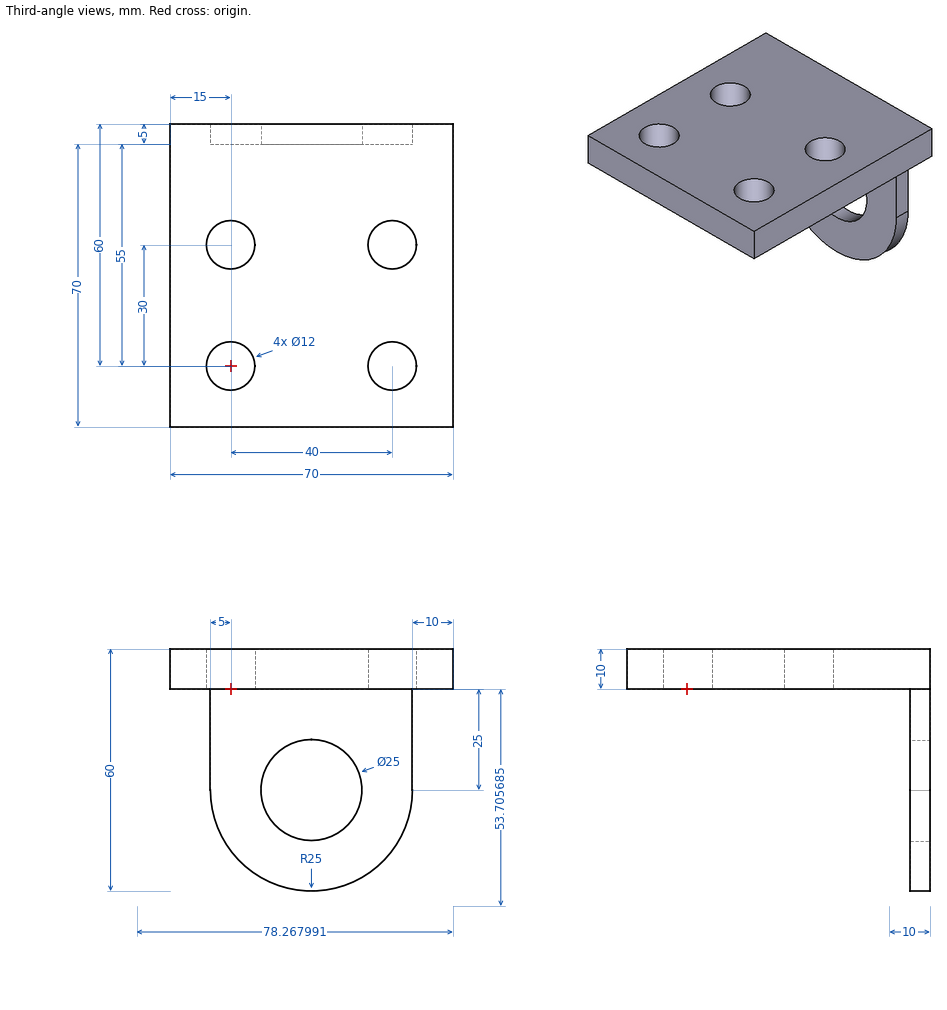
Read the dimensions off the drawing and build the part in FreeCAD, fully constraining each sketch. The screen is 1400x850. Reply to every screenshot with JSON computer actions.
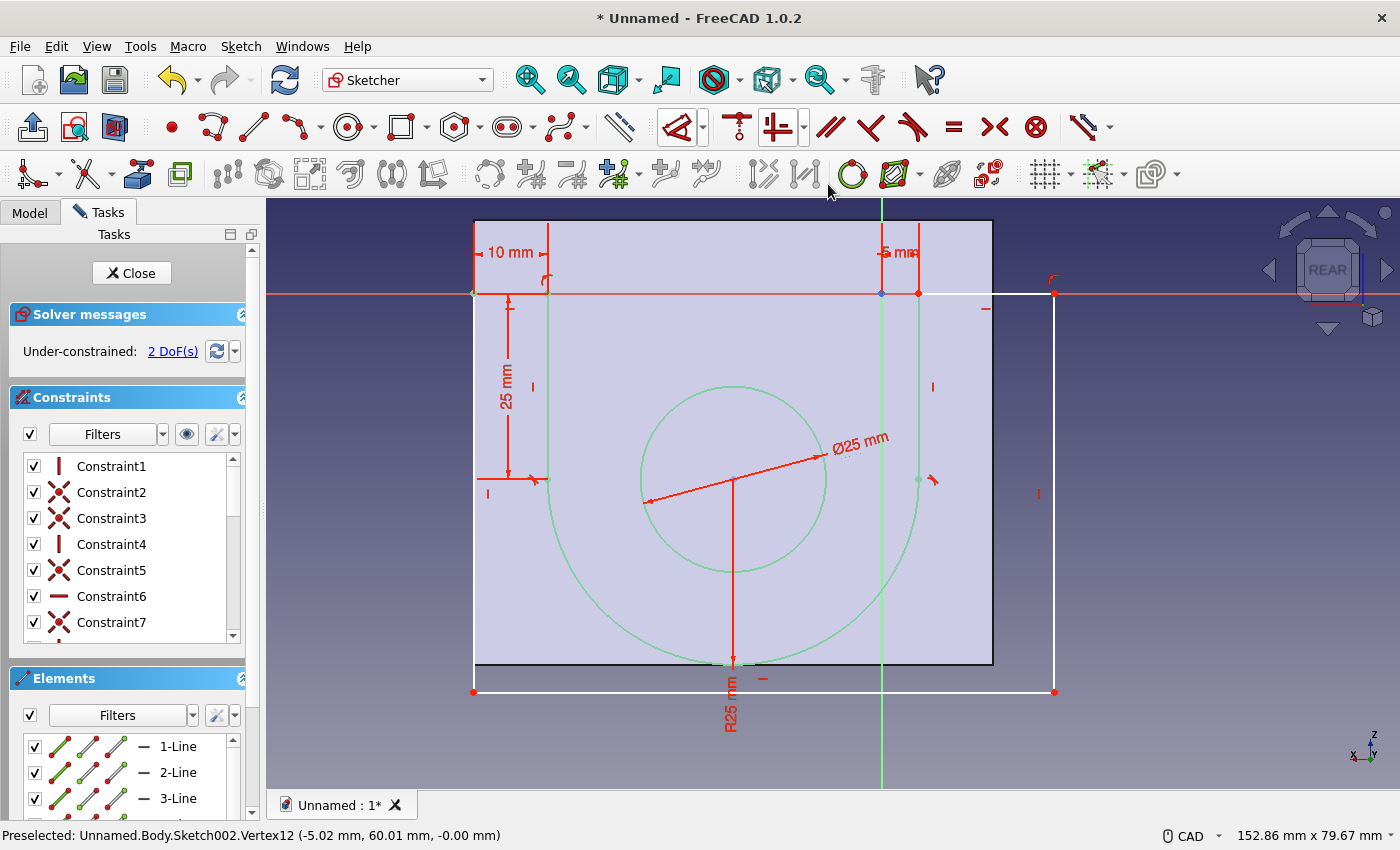
{"action": "left_click", "coordinate": [474, 414]}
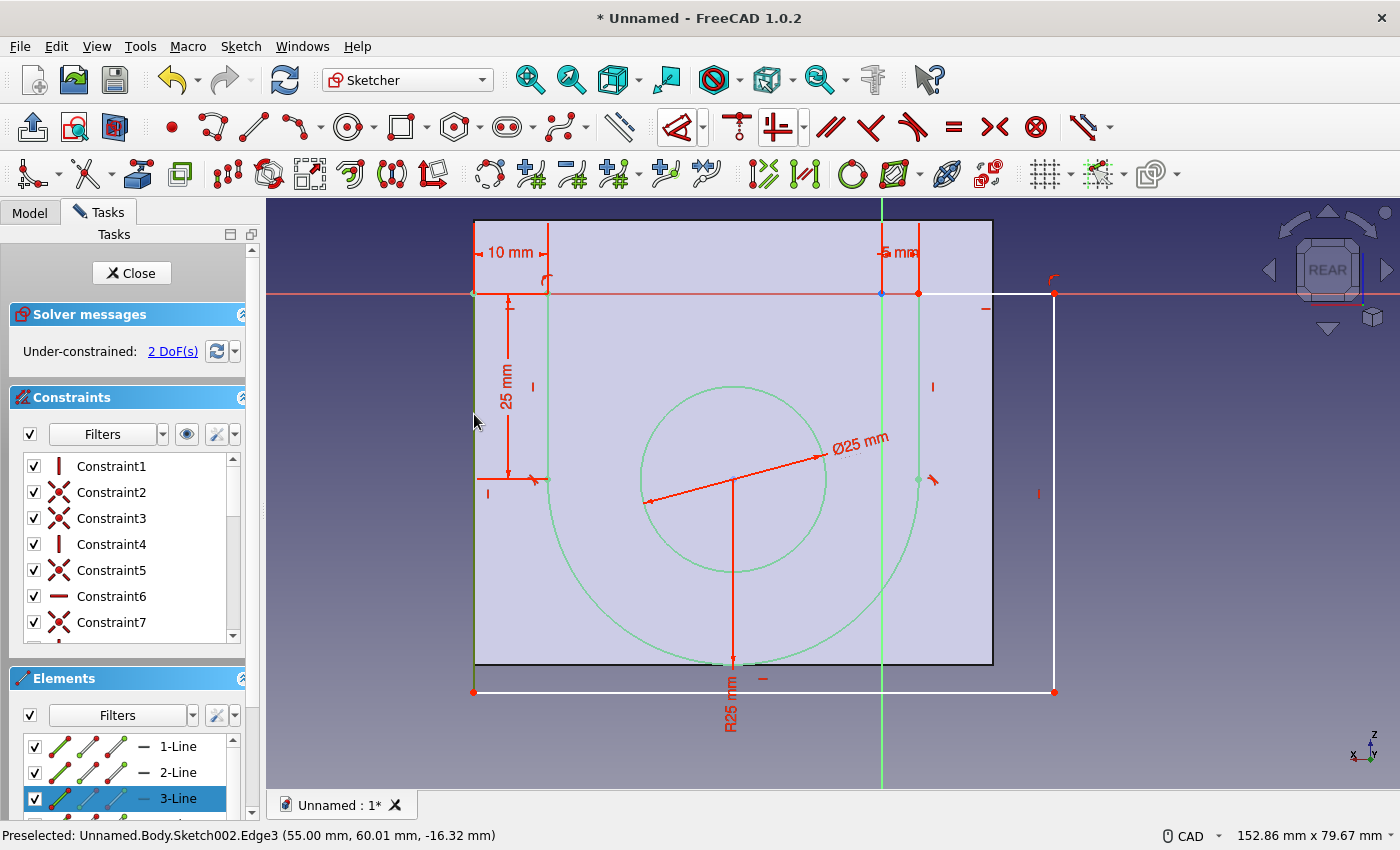
{"action": "key", "text": "i"}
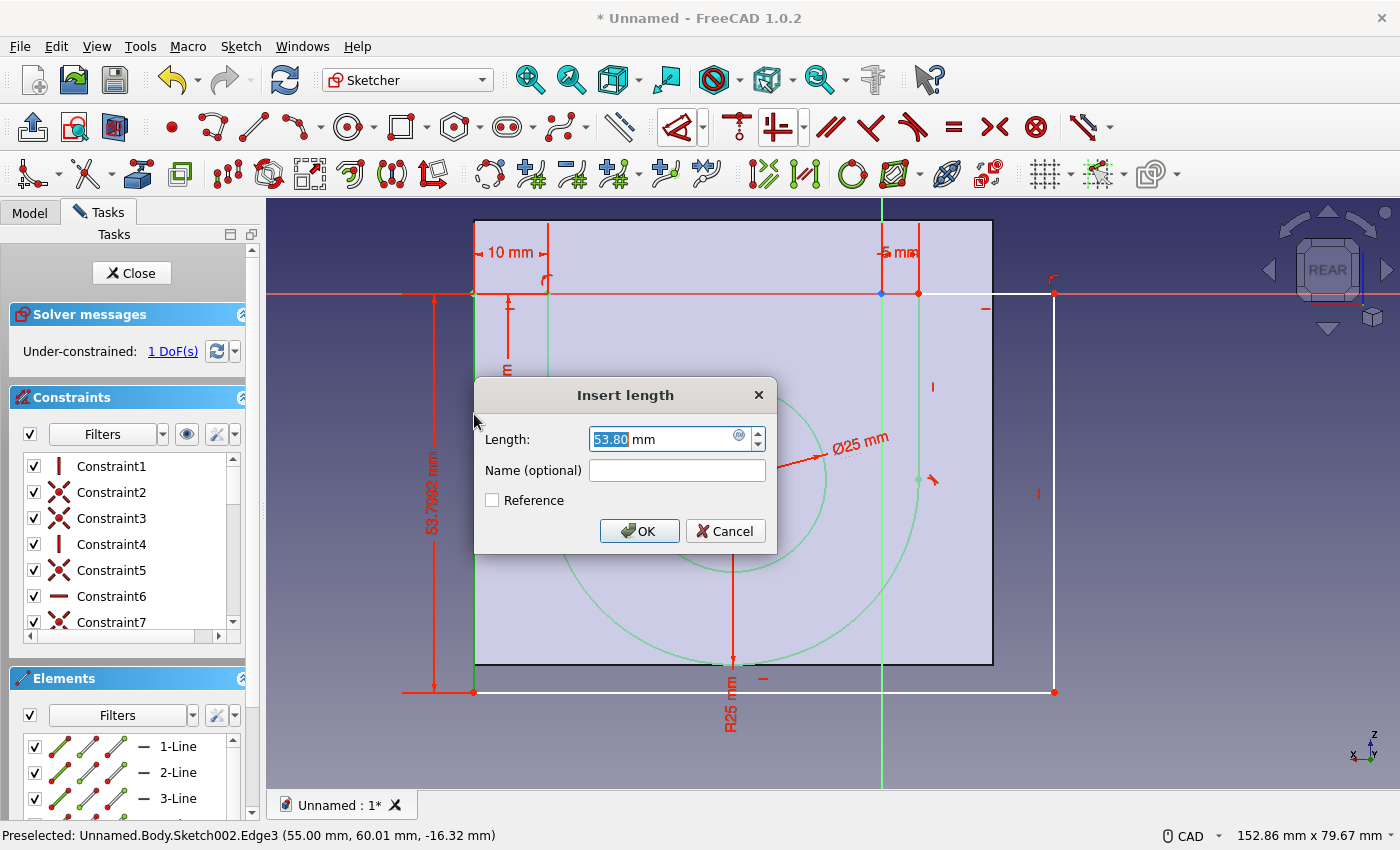
{"action": "type", "text": "53.705685"}
{"action": "key", "text": "Return"}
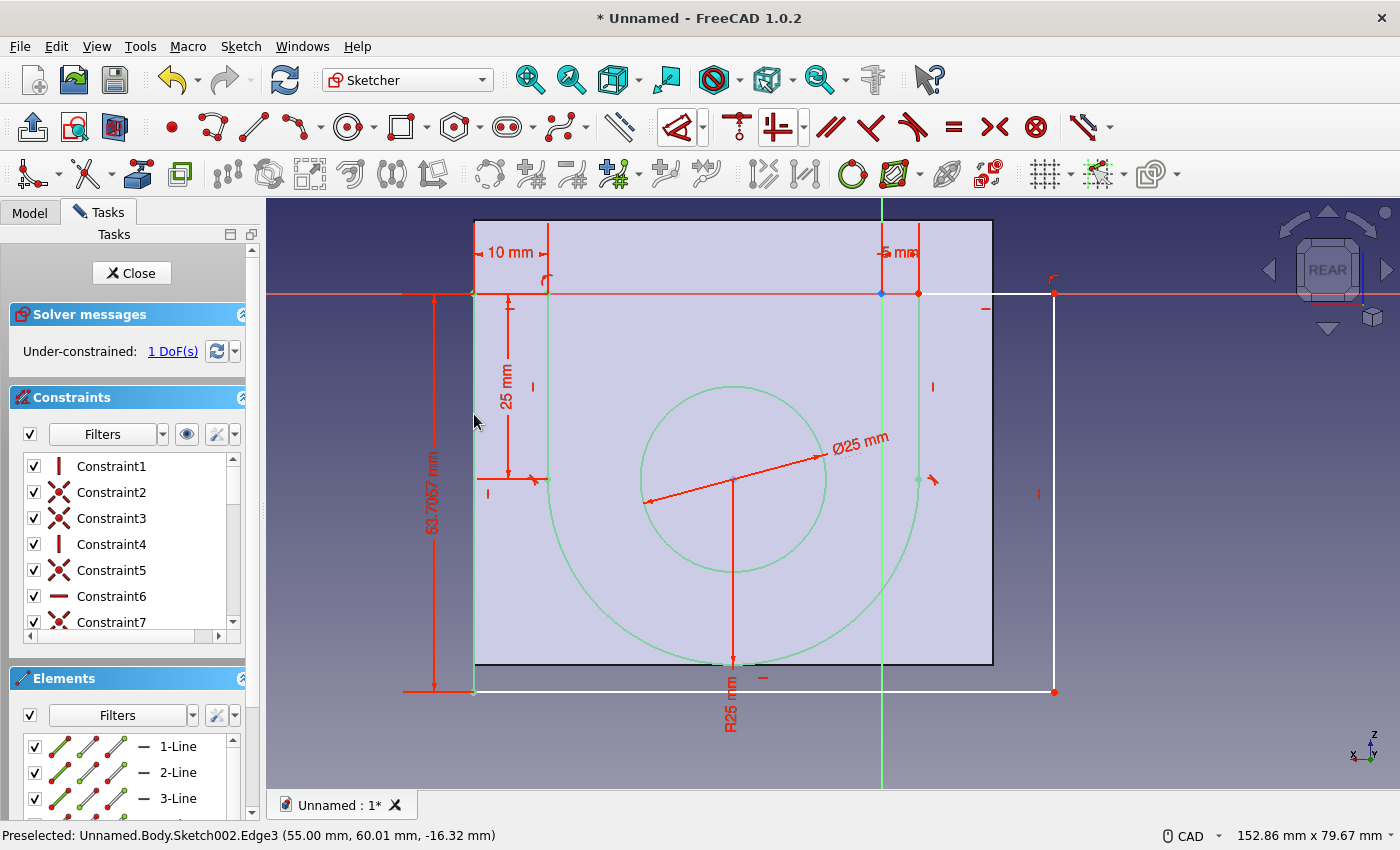
{"action": "left_click", "coordinate": [648, 692]}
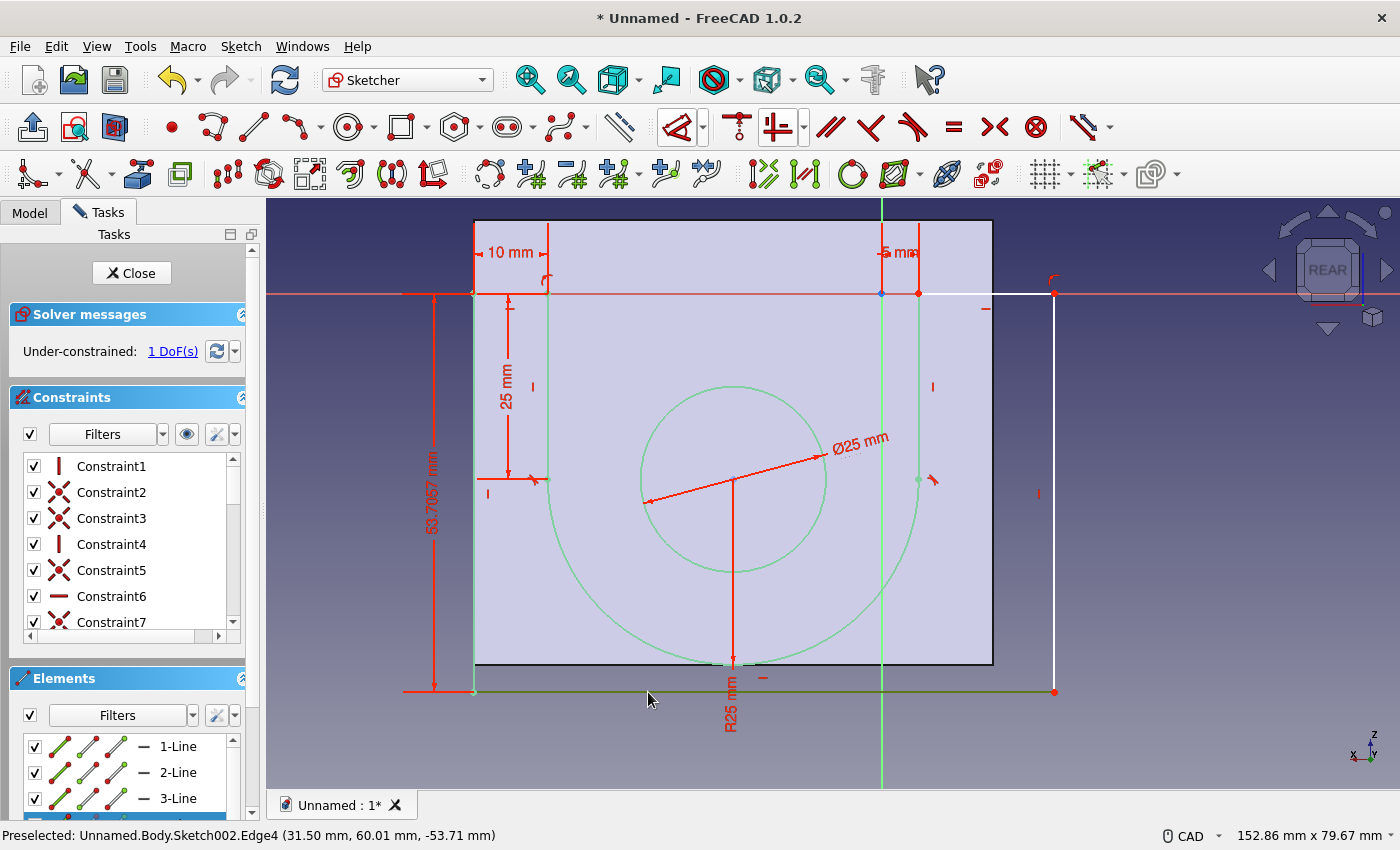
{"action": "key", "text": "l"}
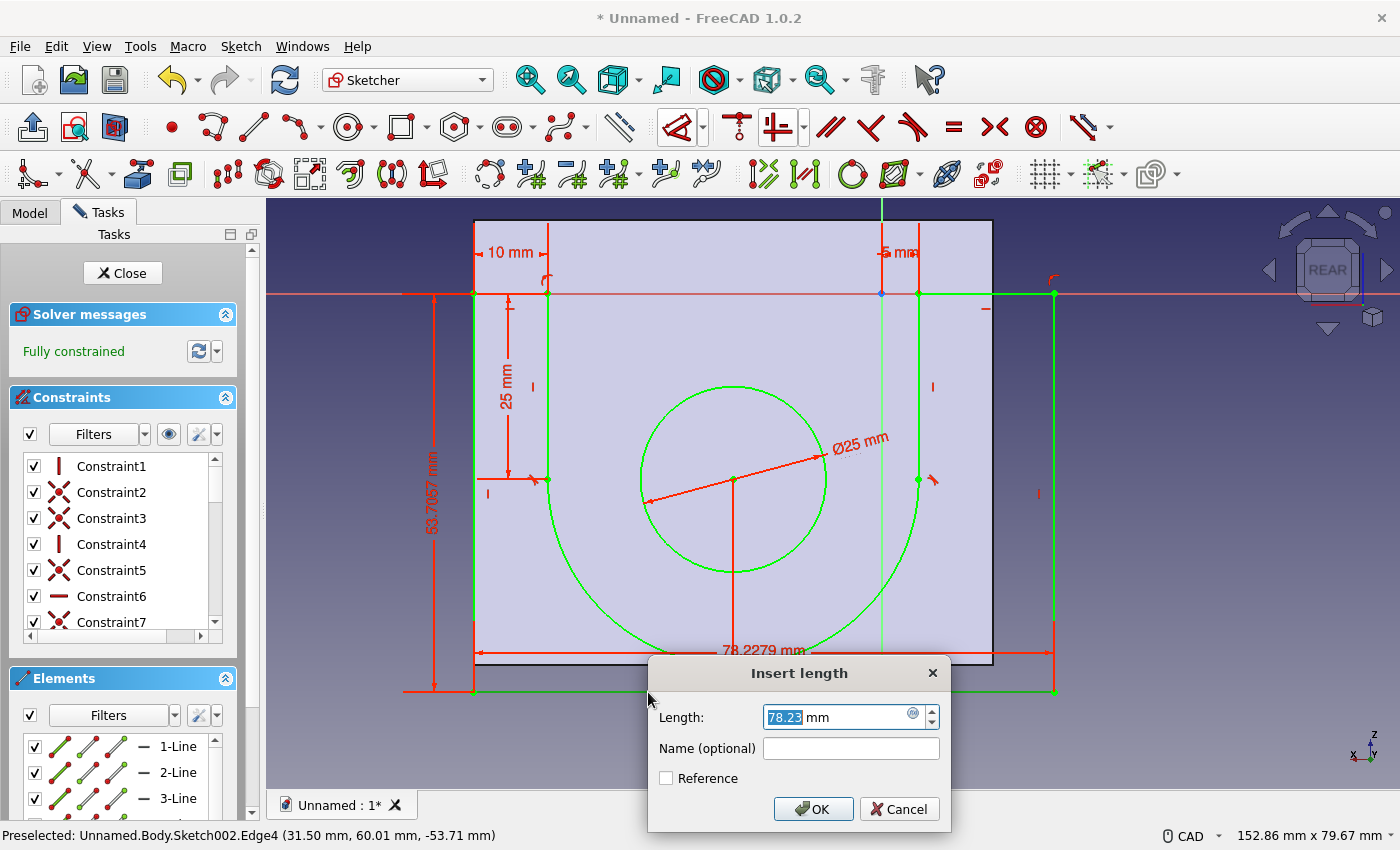
{"action": "type", "text": "78.267991"}
{"action": "key", "text": "Return"}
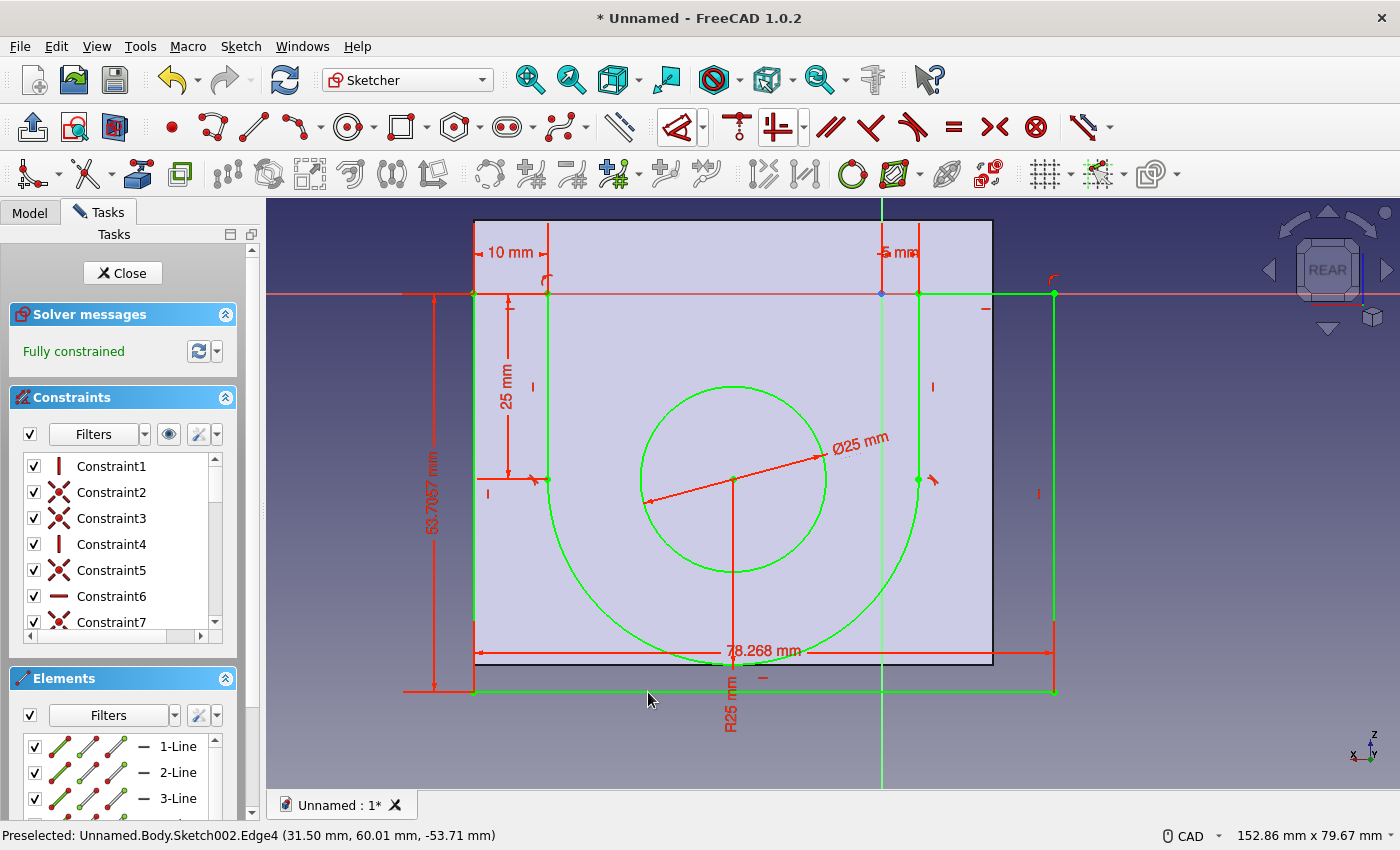
{"action": "left_click", "coordinate": [123, 273]}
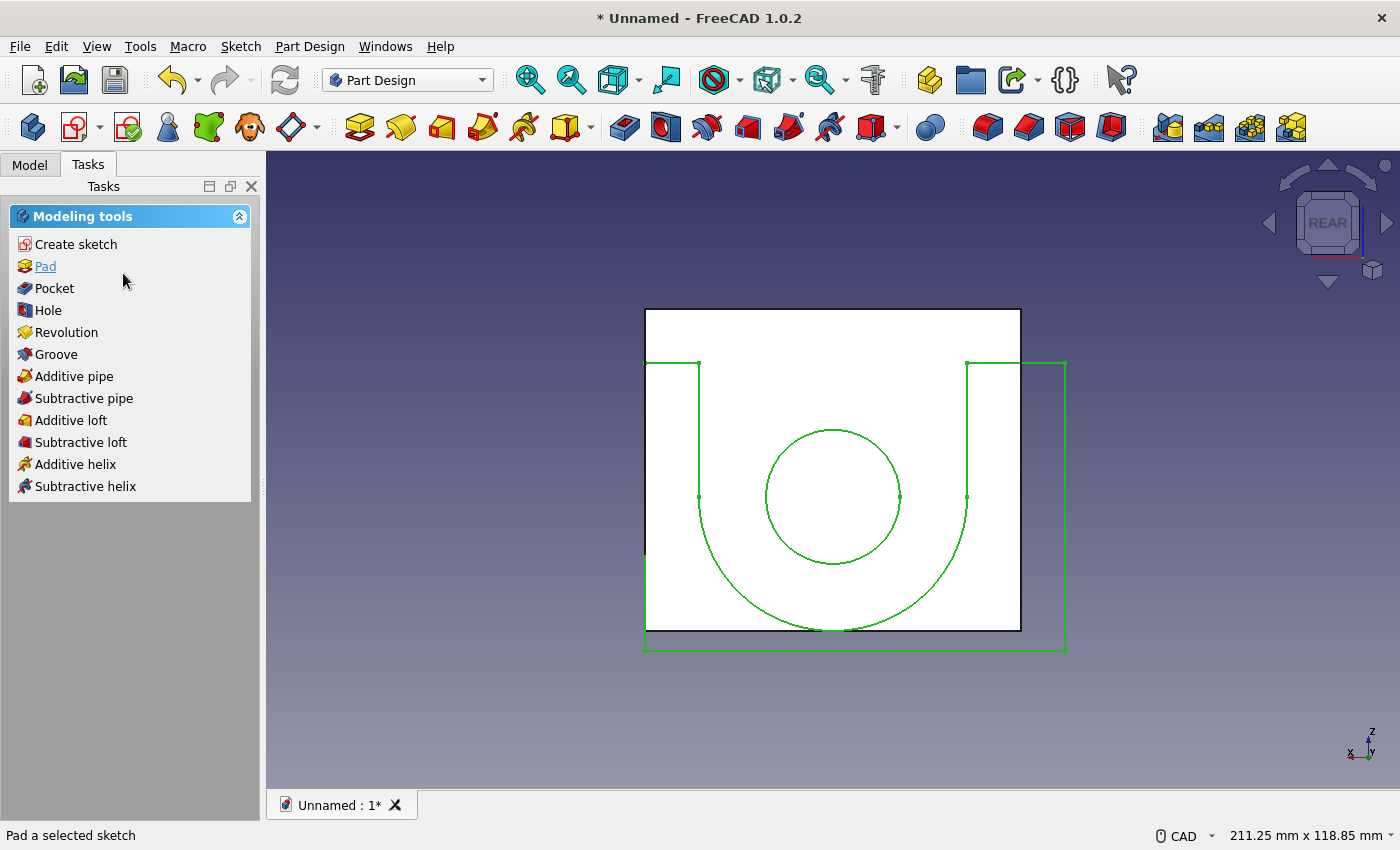
{"action": "left_click", "coordinate": [625, 128]}